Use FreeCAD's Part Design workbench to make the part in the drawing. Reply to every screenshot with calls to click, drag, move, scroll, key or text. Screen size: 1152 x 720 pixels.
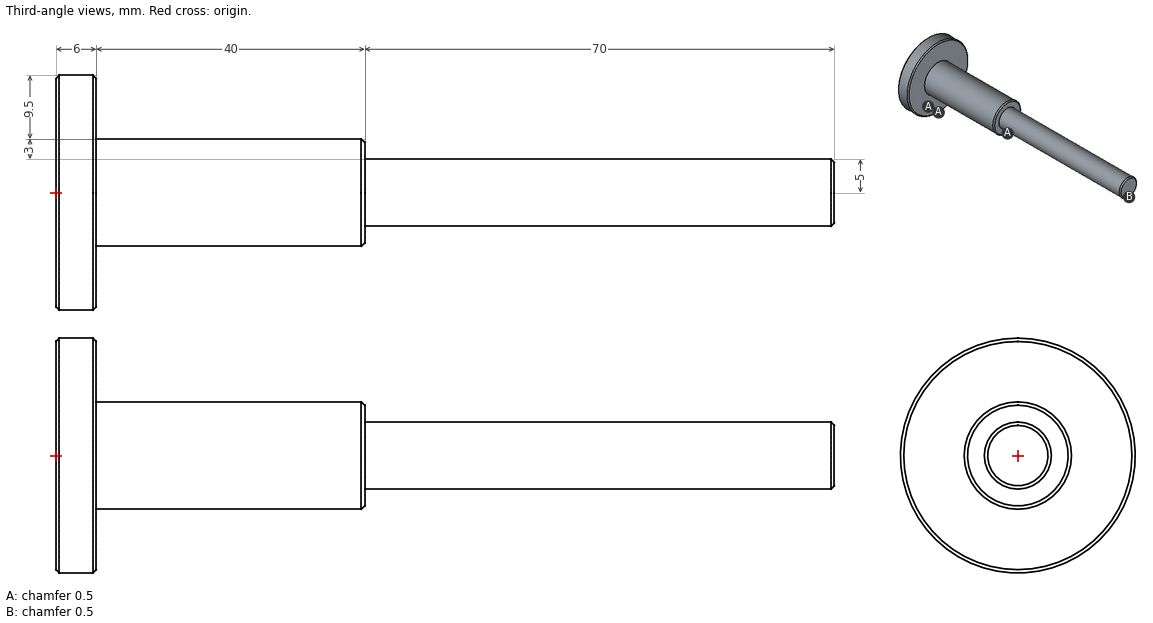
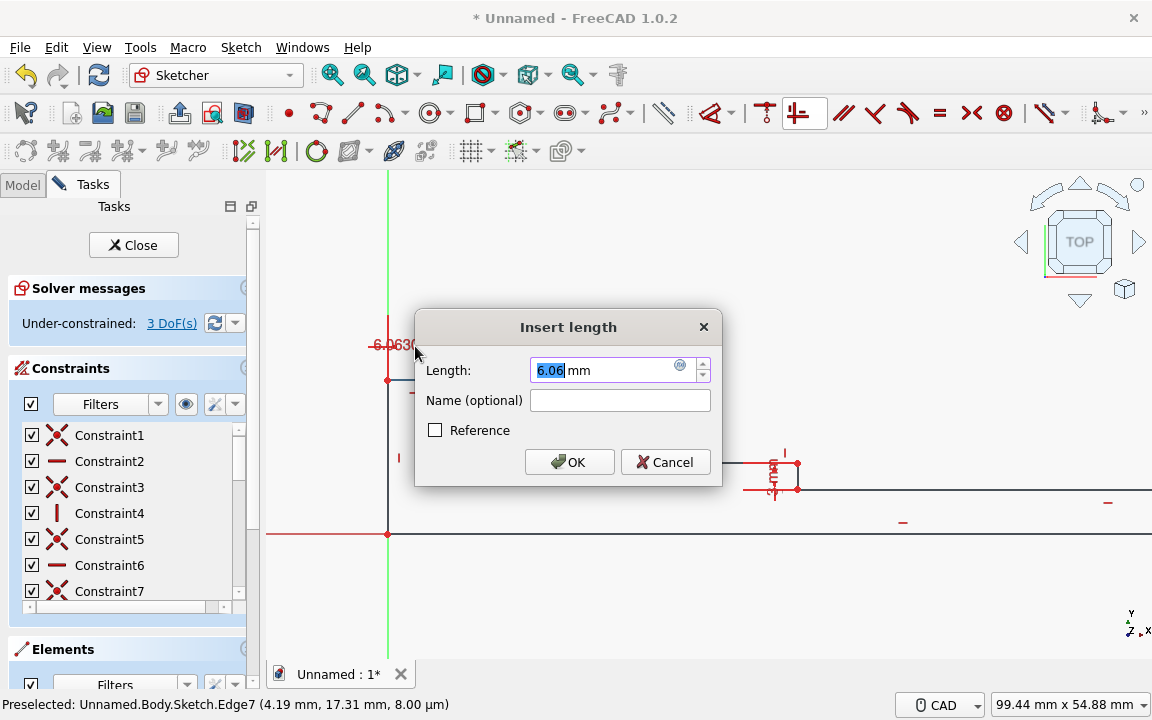
text(6)
key(Return)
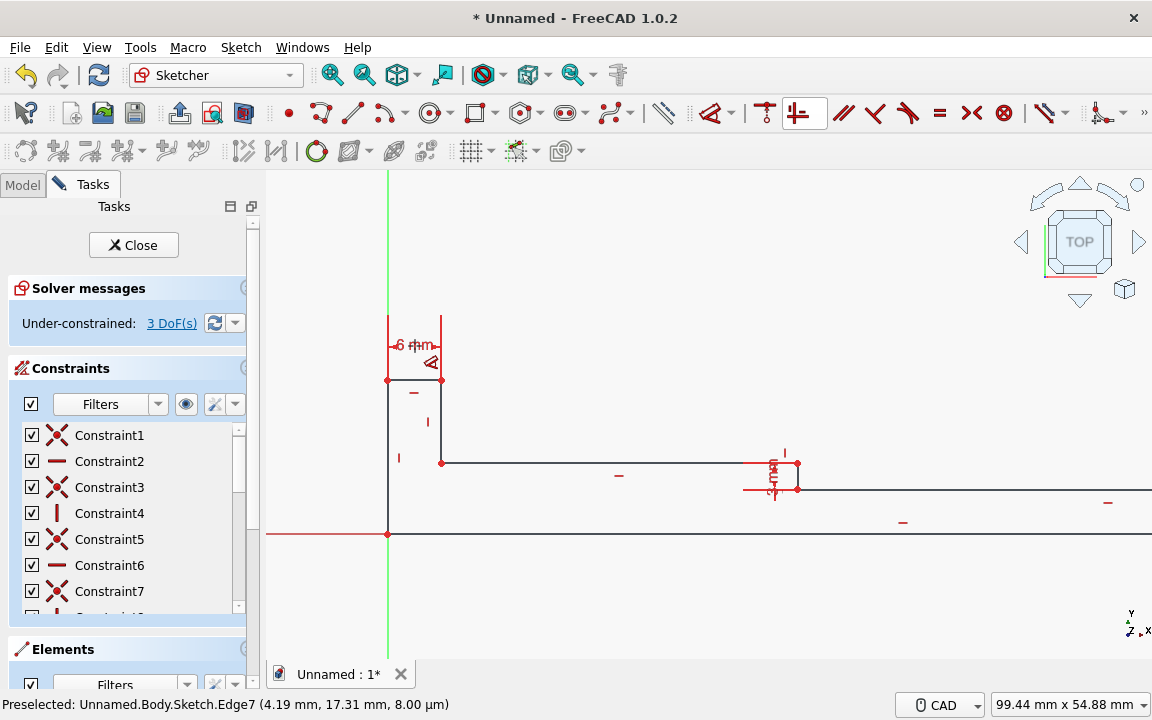
click(984, 490)
click(892, 456)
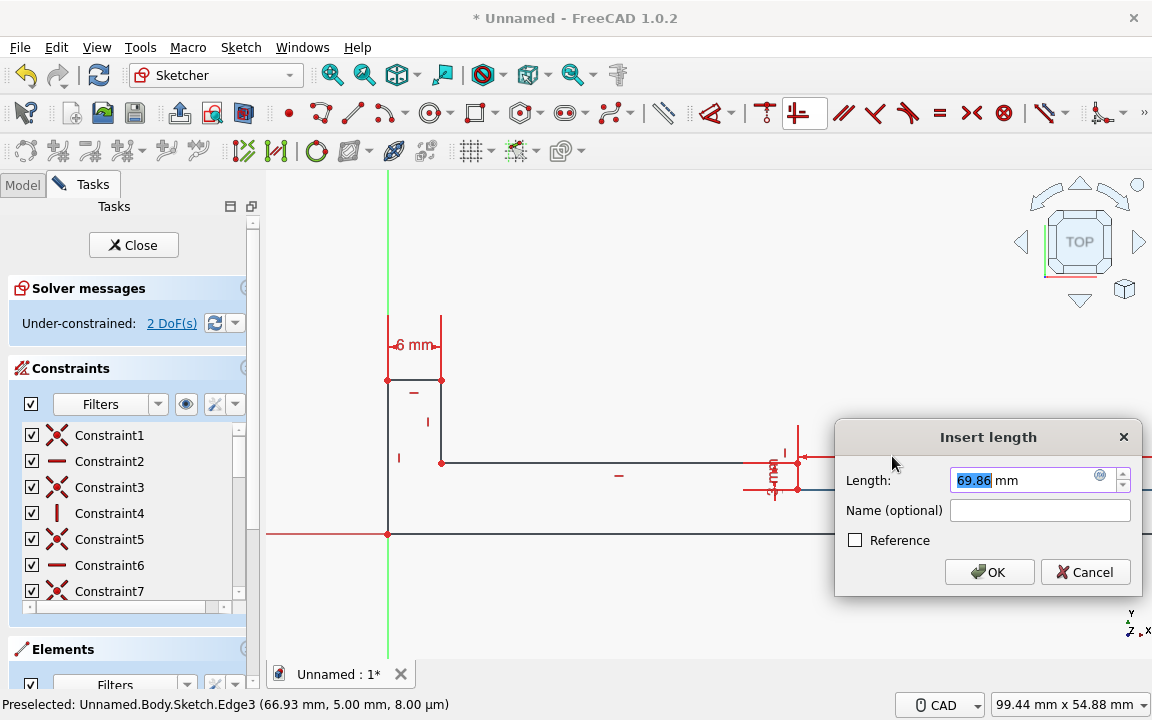
text(70)
key(Return)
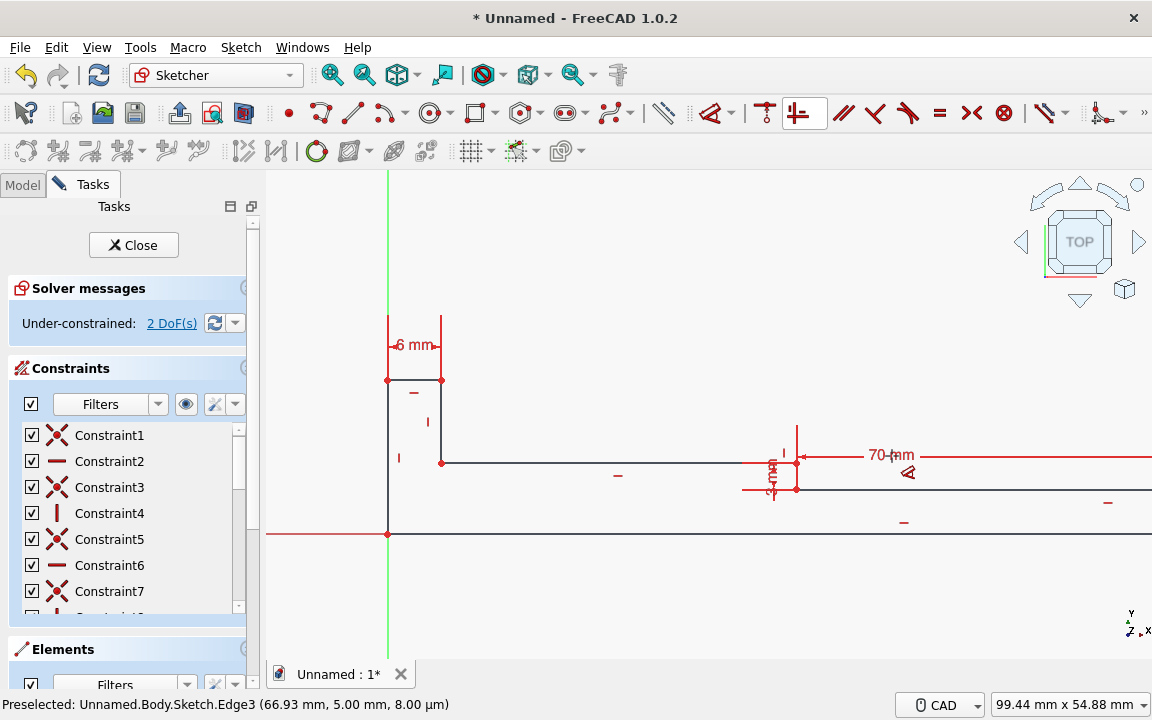
click(690, 463)
click(619, 497)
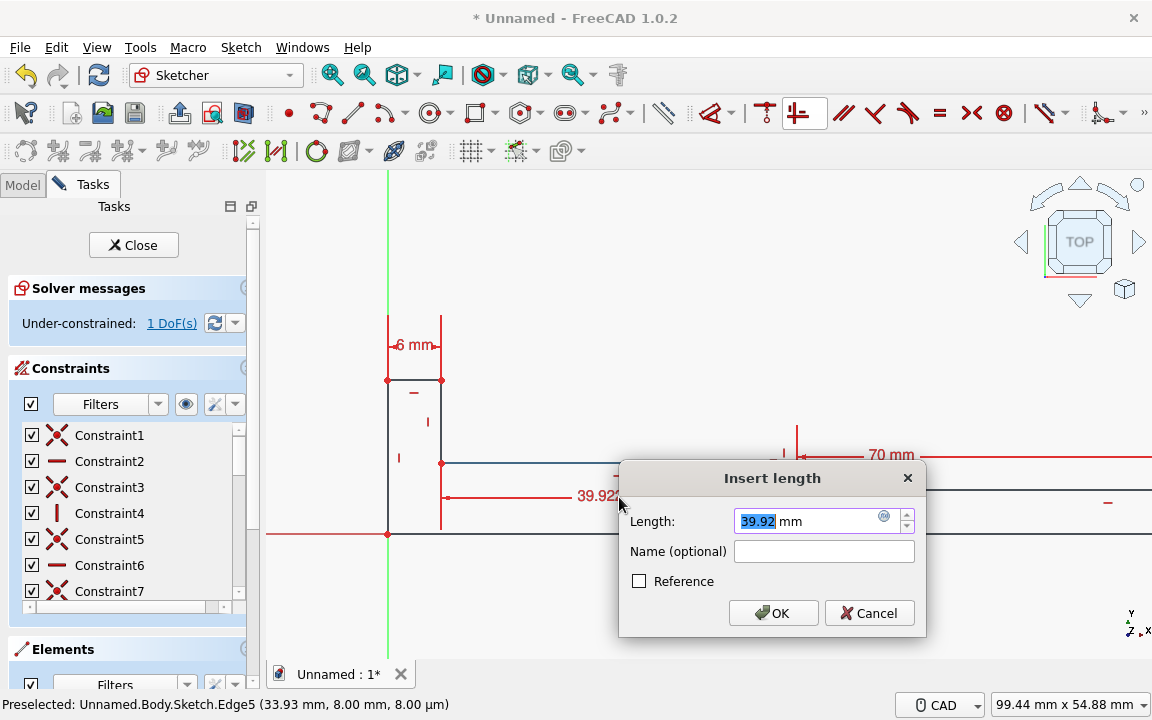
text(40)
key(Return)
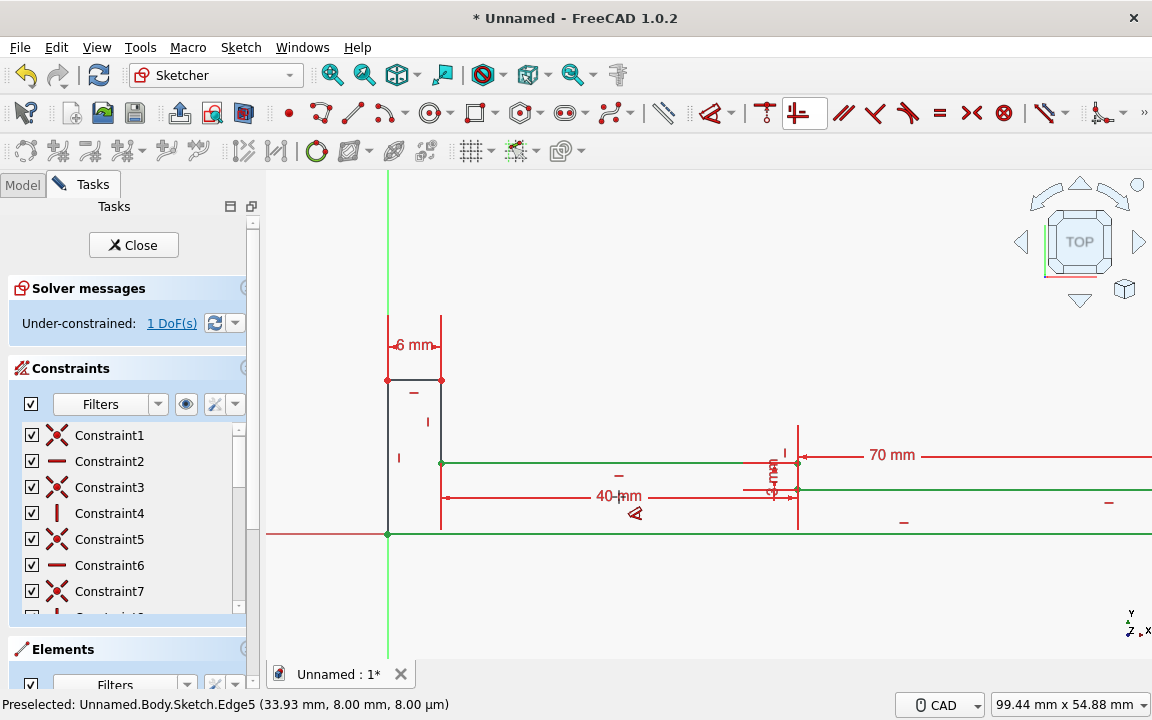
click(441, 438)
click(407, 422)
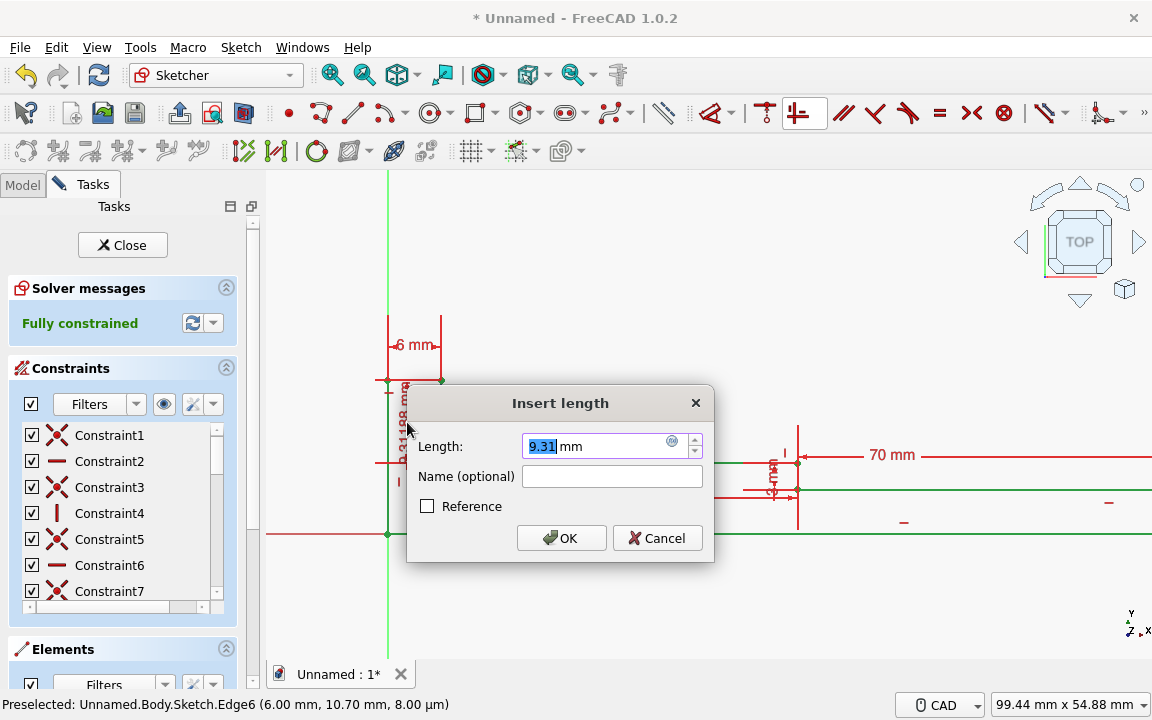
text(9.5)
key(Return)
key(Escape)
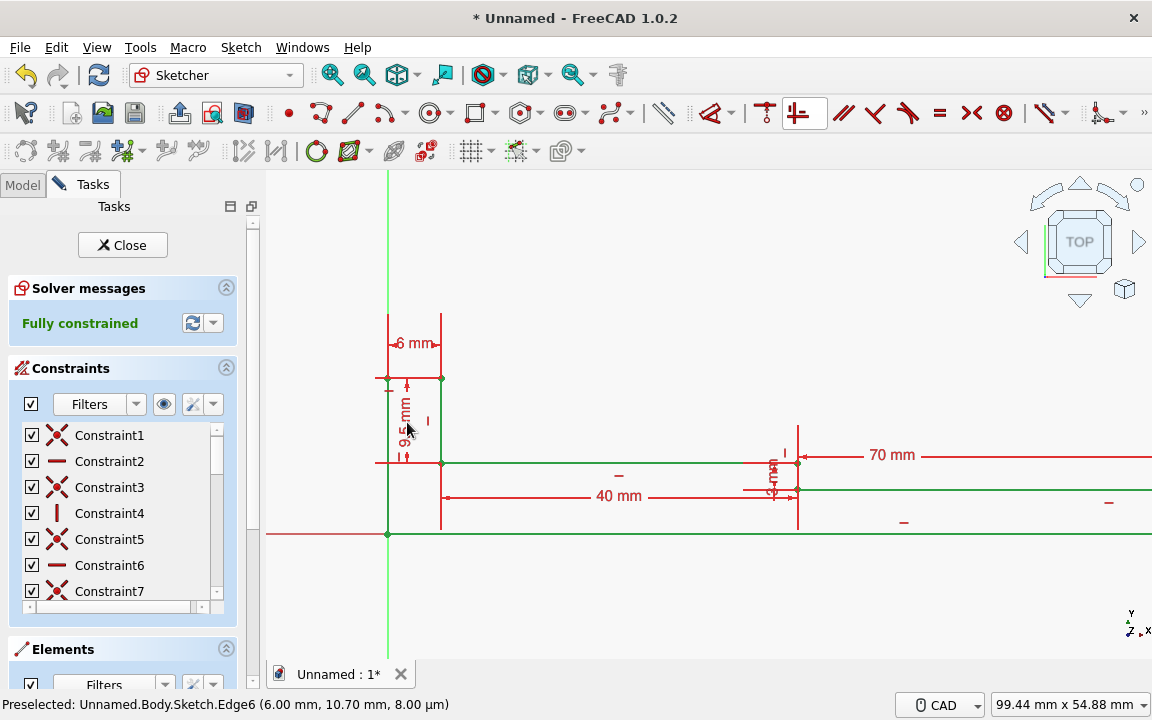
click(123, 245)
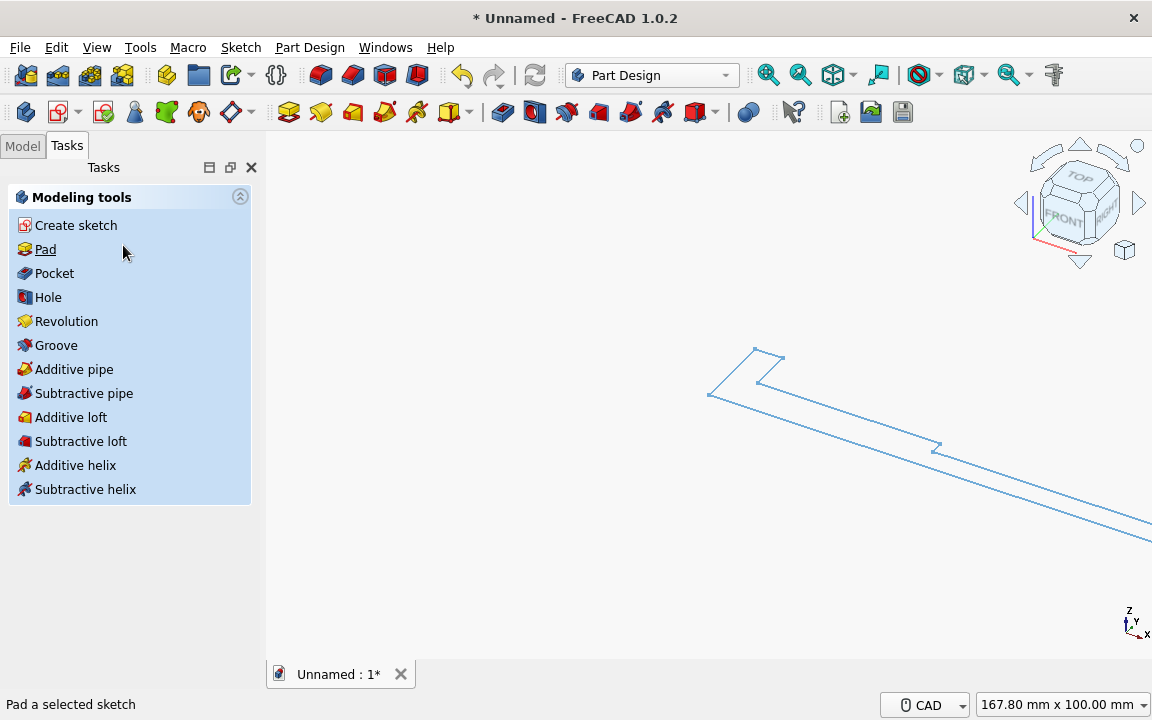
click(322, 112)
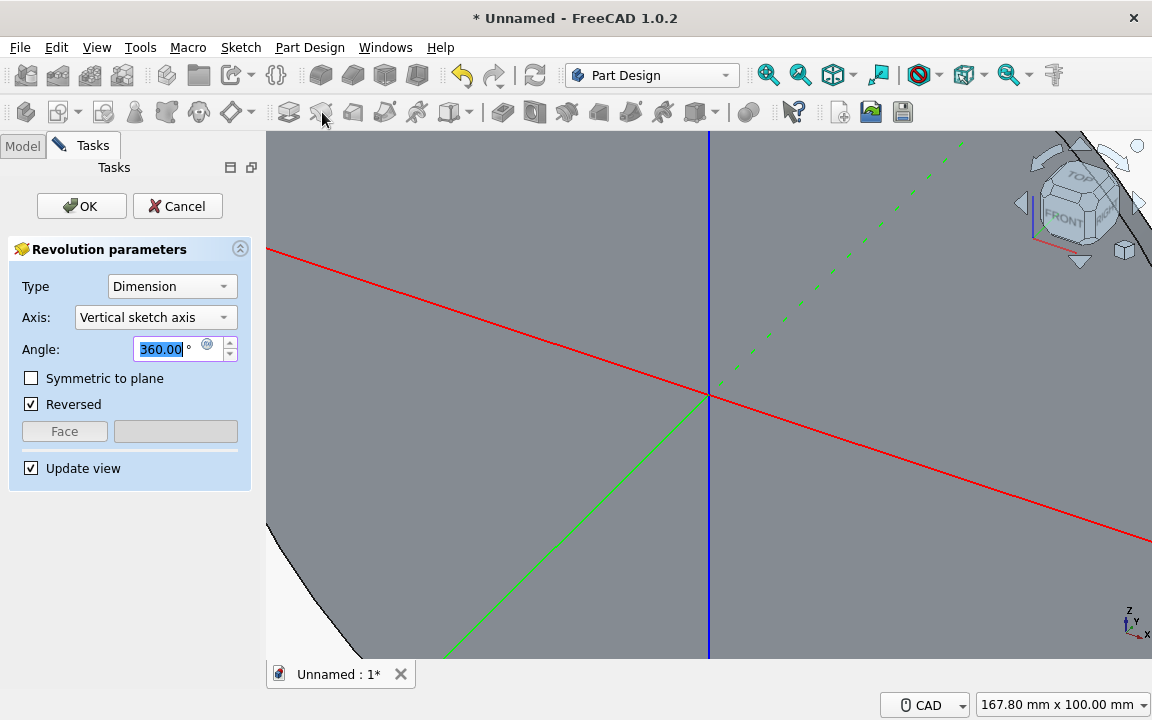
click(156, 318)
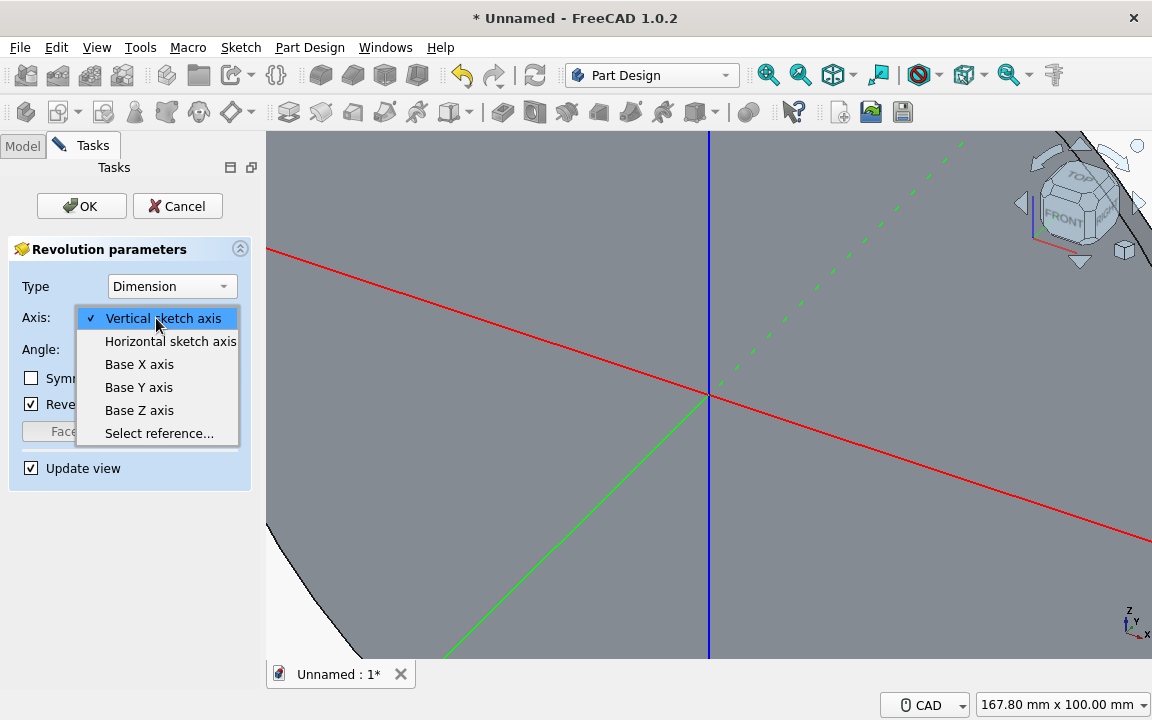
click(156, 342)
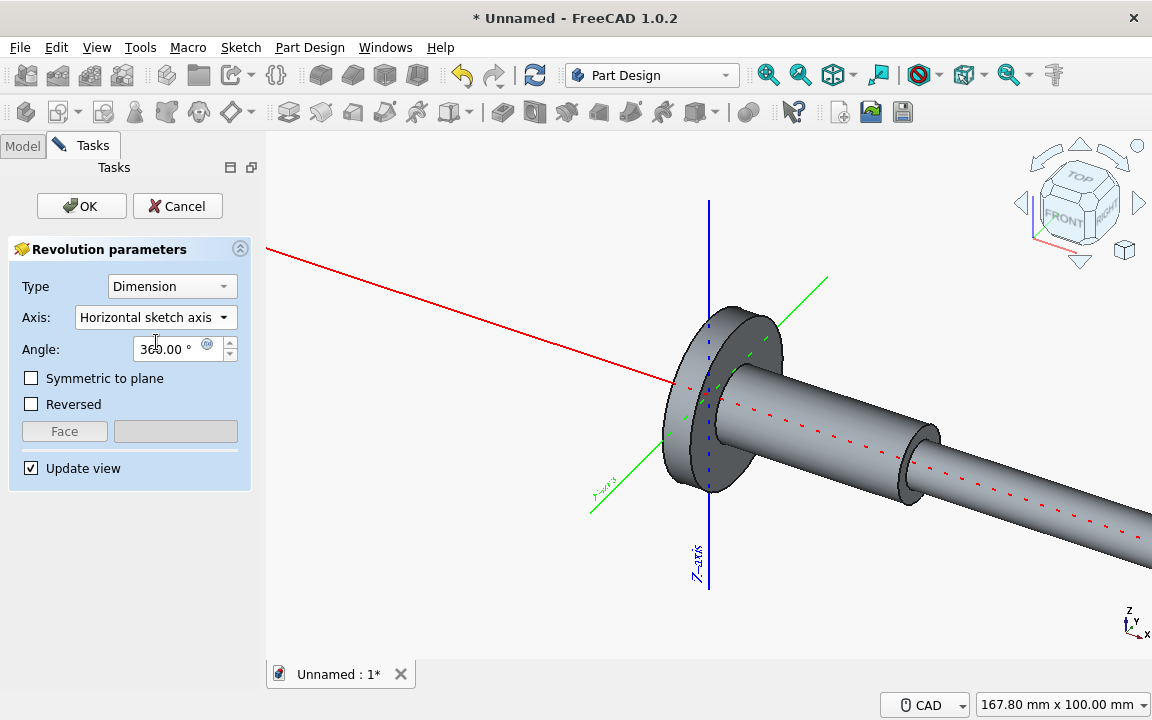
click(82, 206)